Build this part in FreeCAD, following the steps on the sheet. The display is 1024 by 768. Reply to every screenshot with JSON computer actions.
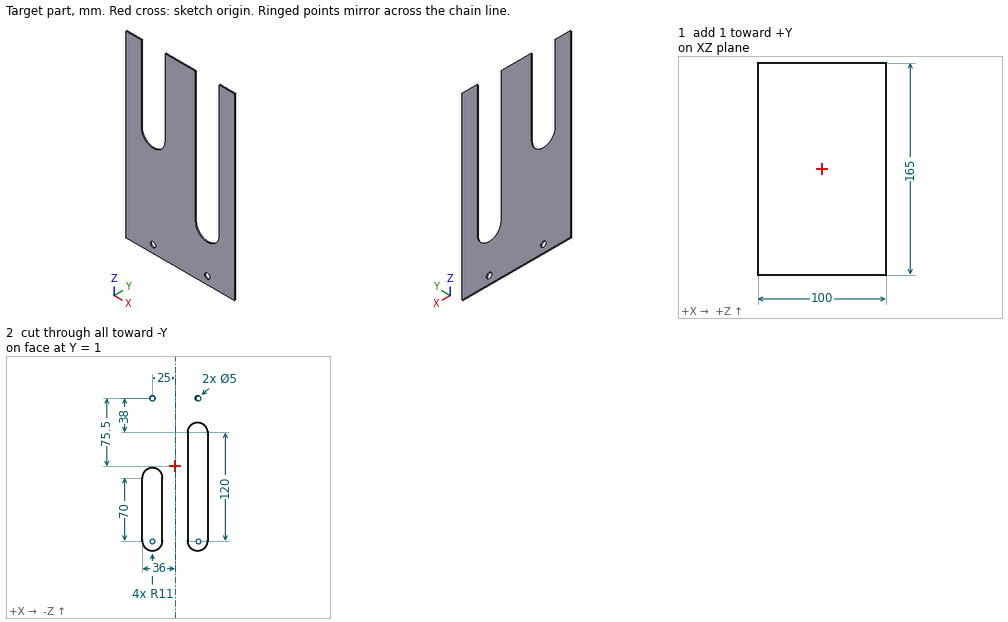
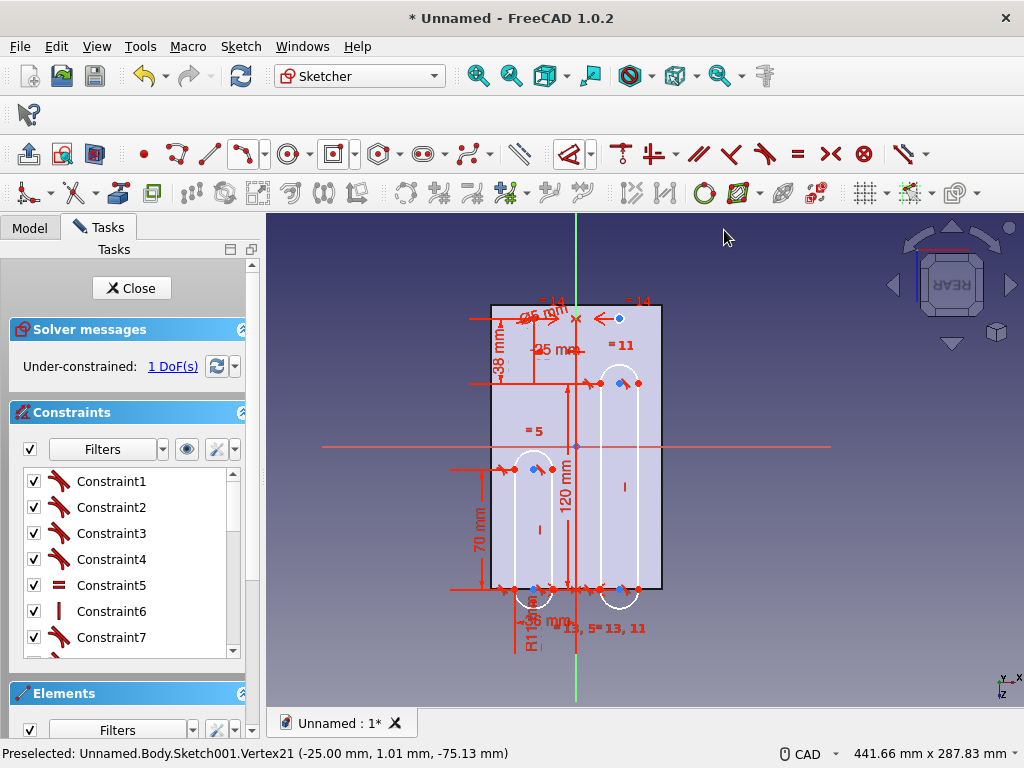
{"action": "left_click", "coordinate": [534, 319]}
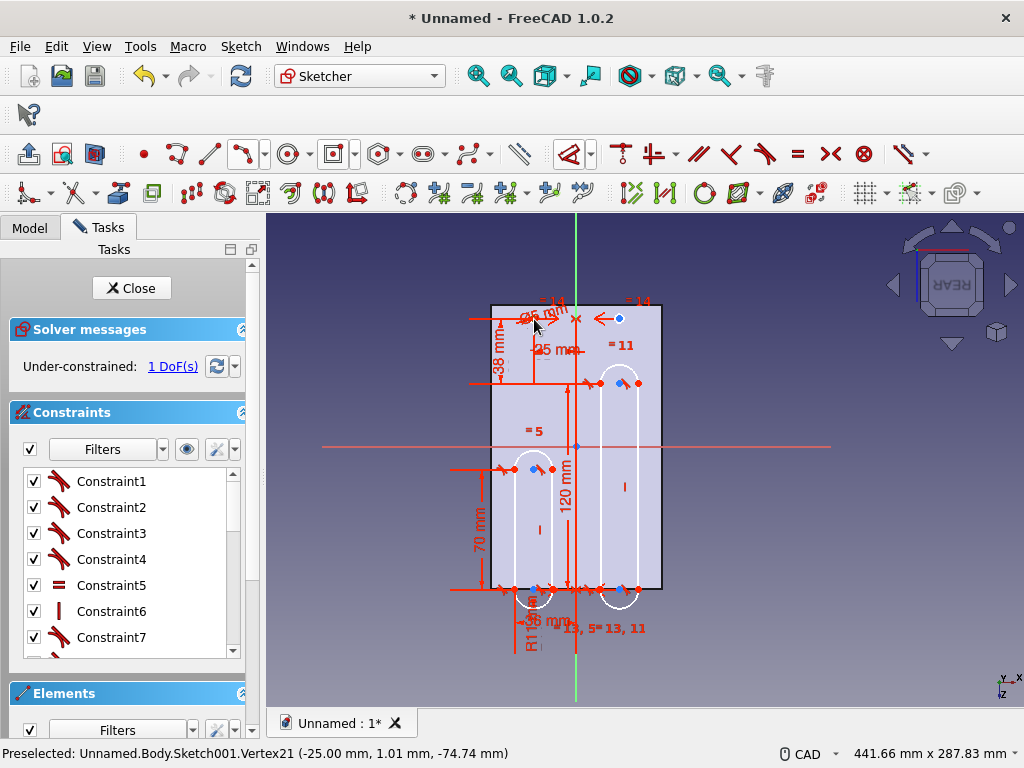
{"action": "key", "text": "i"}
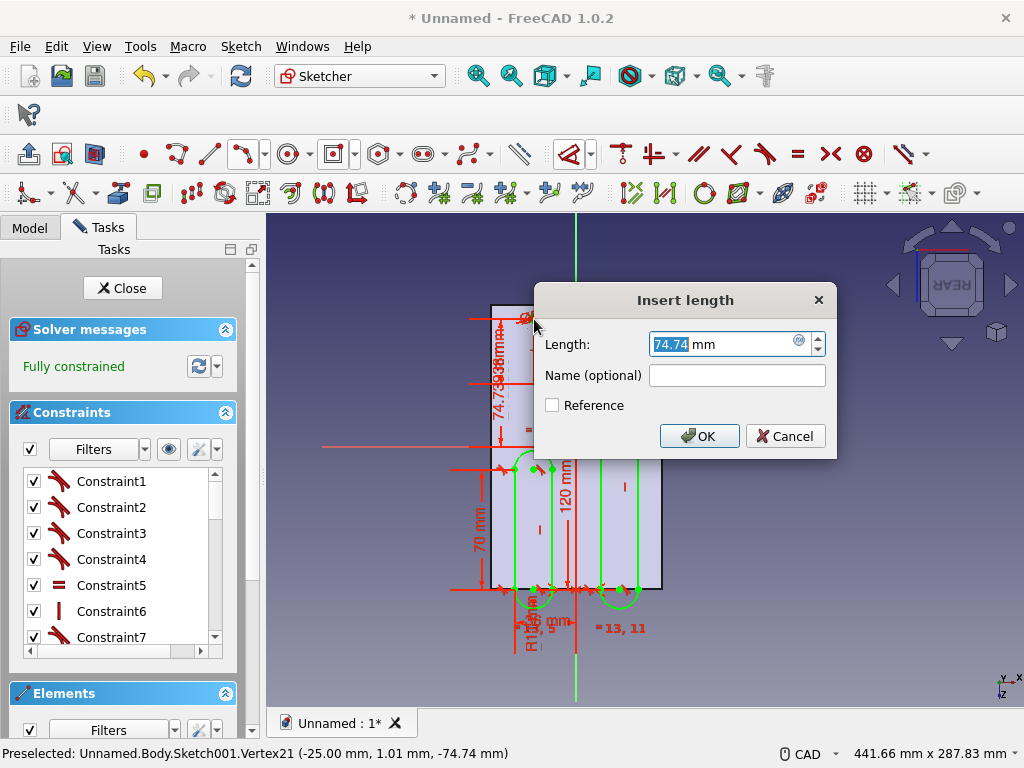
{"action": "type", "text": "75.5"}
{"action": "key", "text": "Return"}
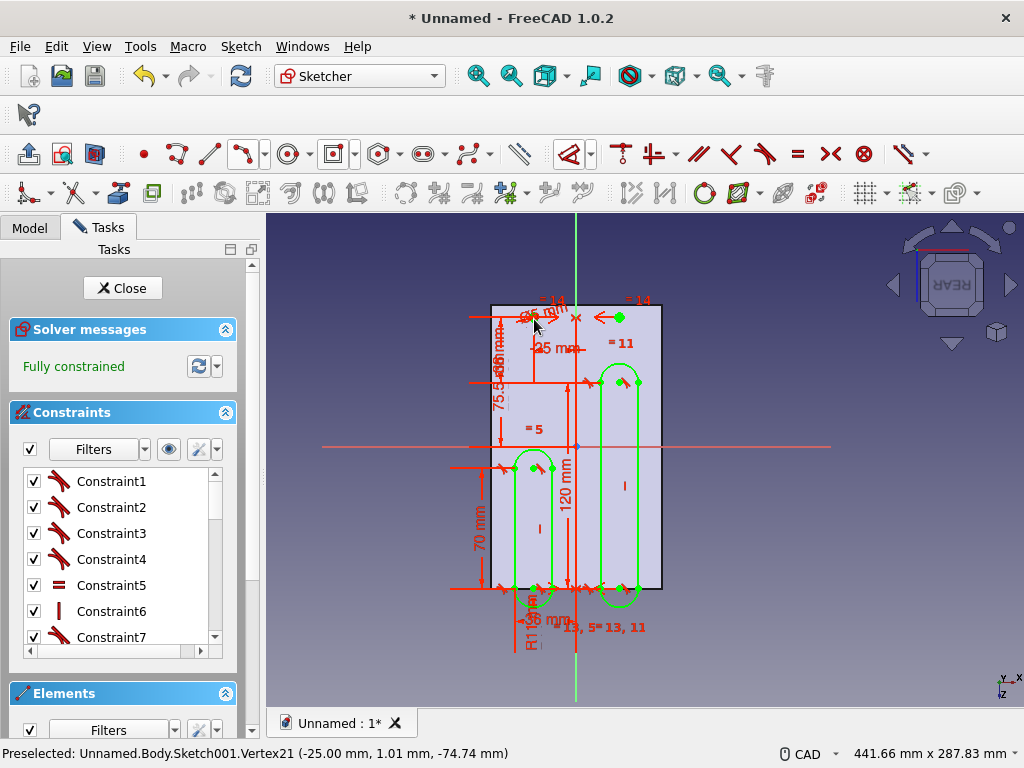
{"action": "left_click", "coordinate": [123, 288]}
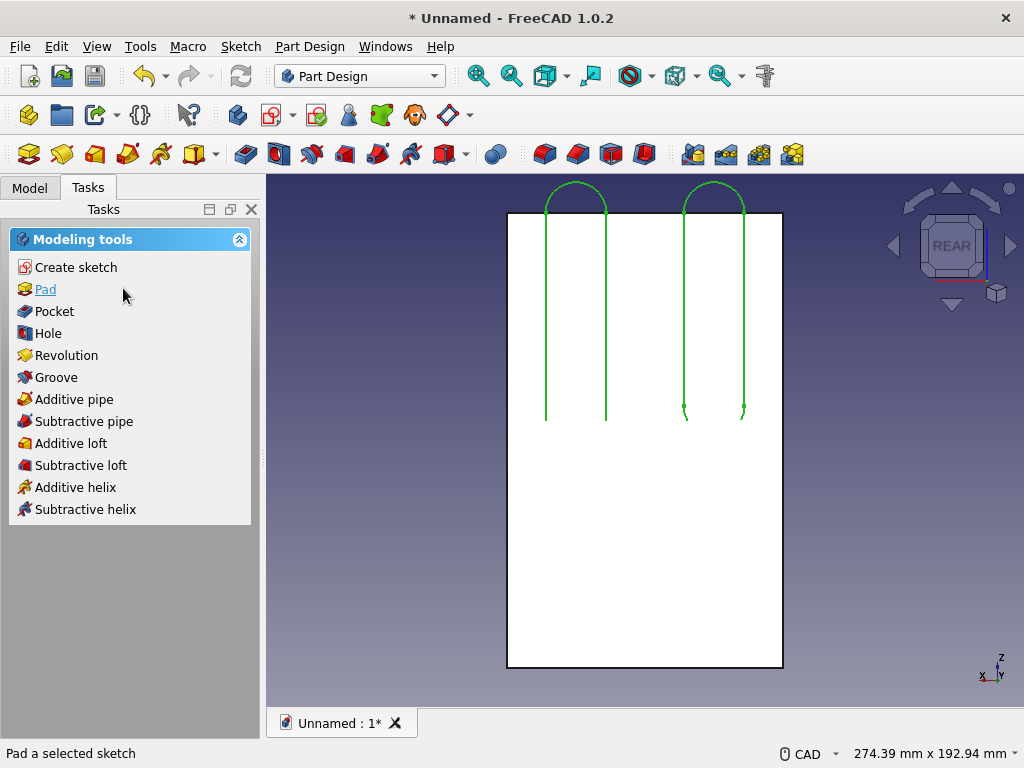
{"action": "left_click", "coordinate": [246, 154]}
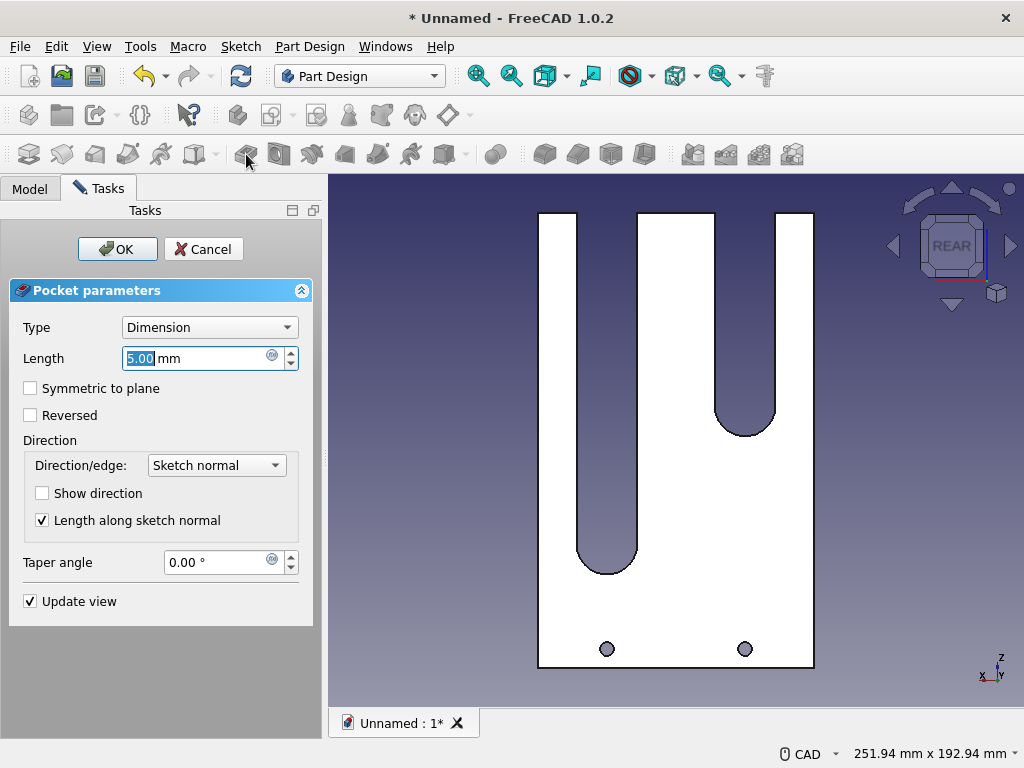
{"action": "left_click", "coordinate": [210, 328]}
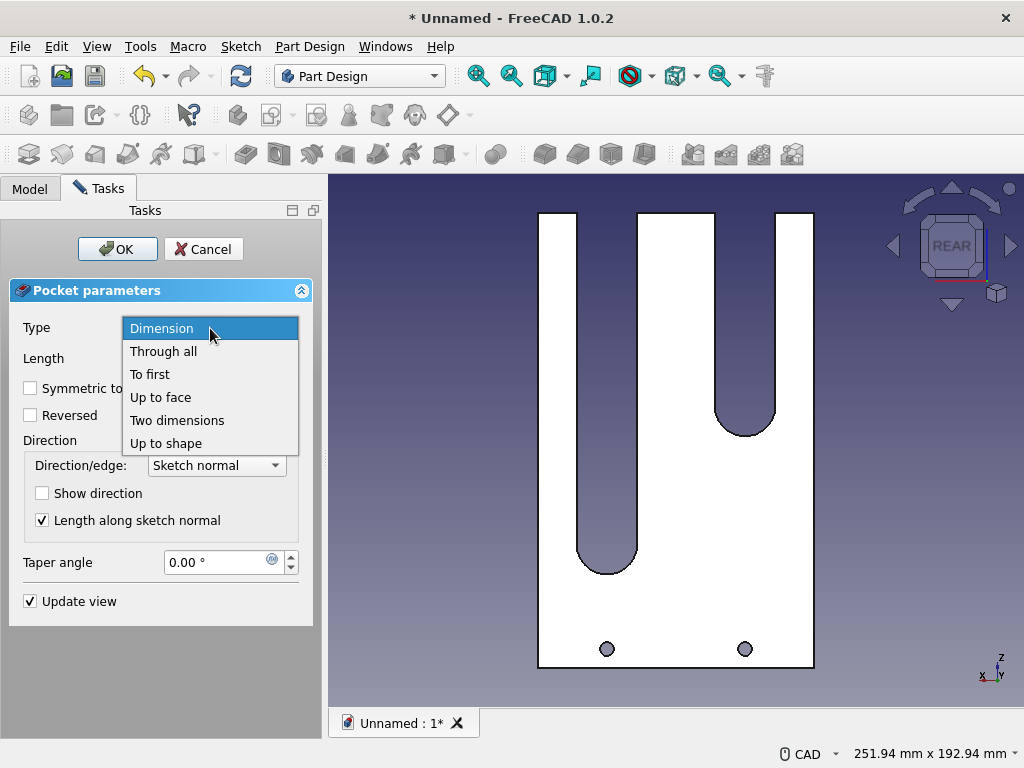
{"action": "left_click", "coordinate": [208, 352]}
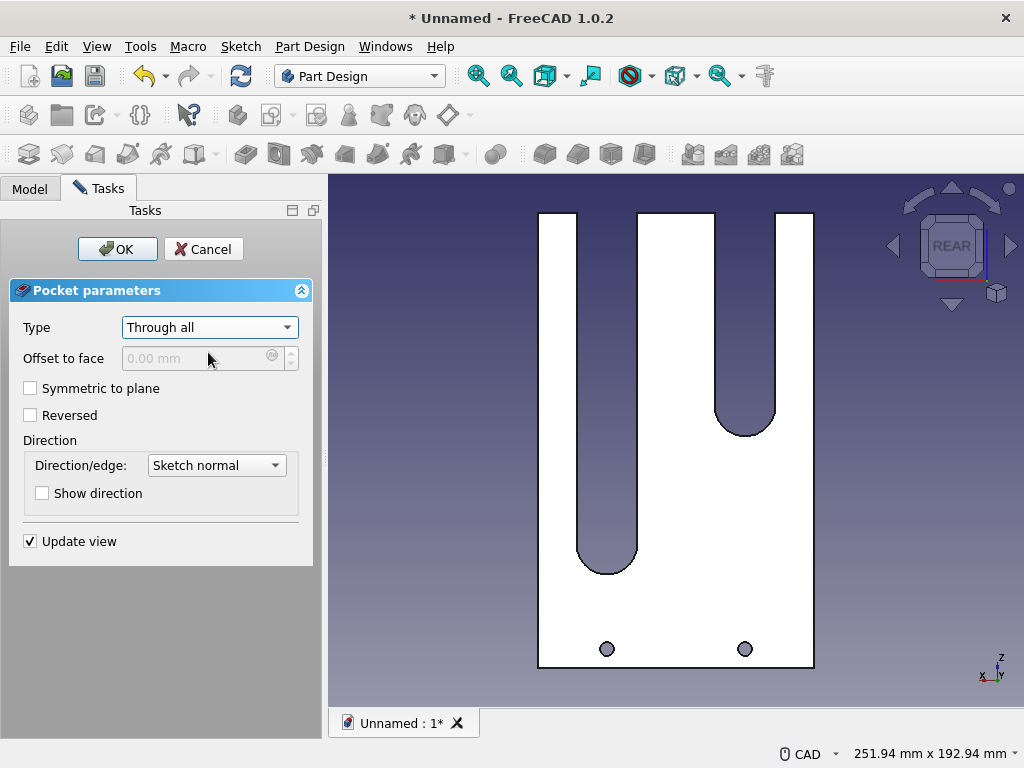
{"action": "left_click", "coordinate": [118, 249]}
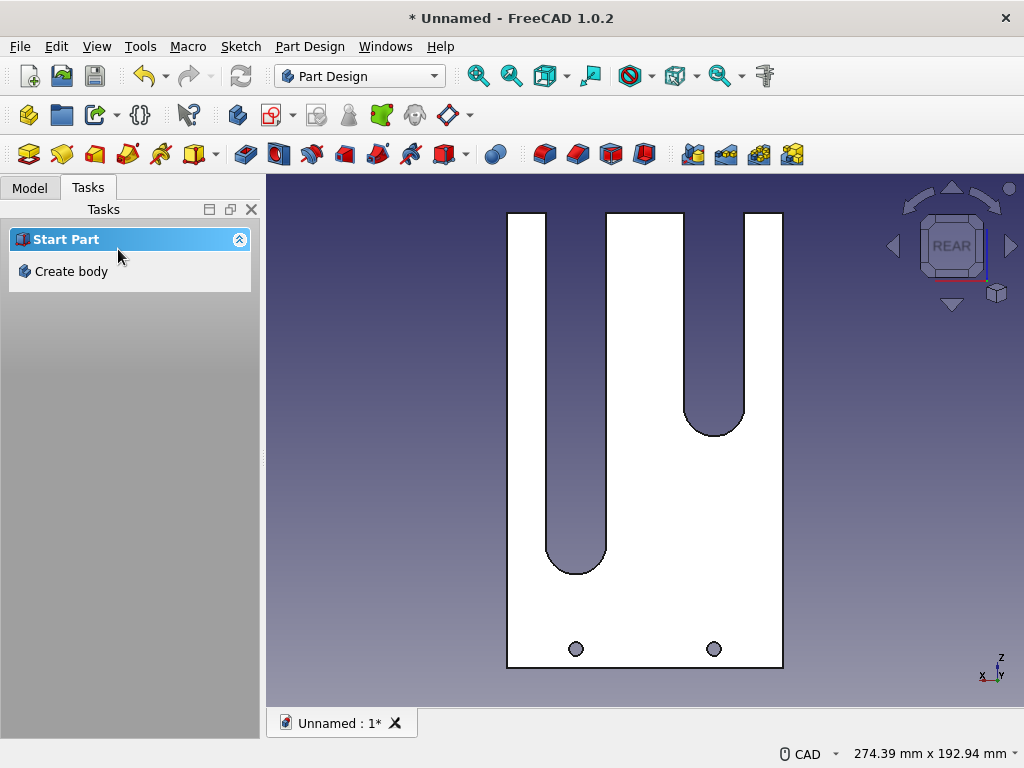
{"action": "key", "text": "0"}